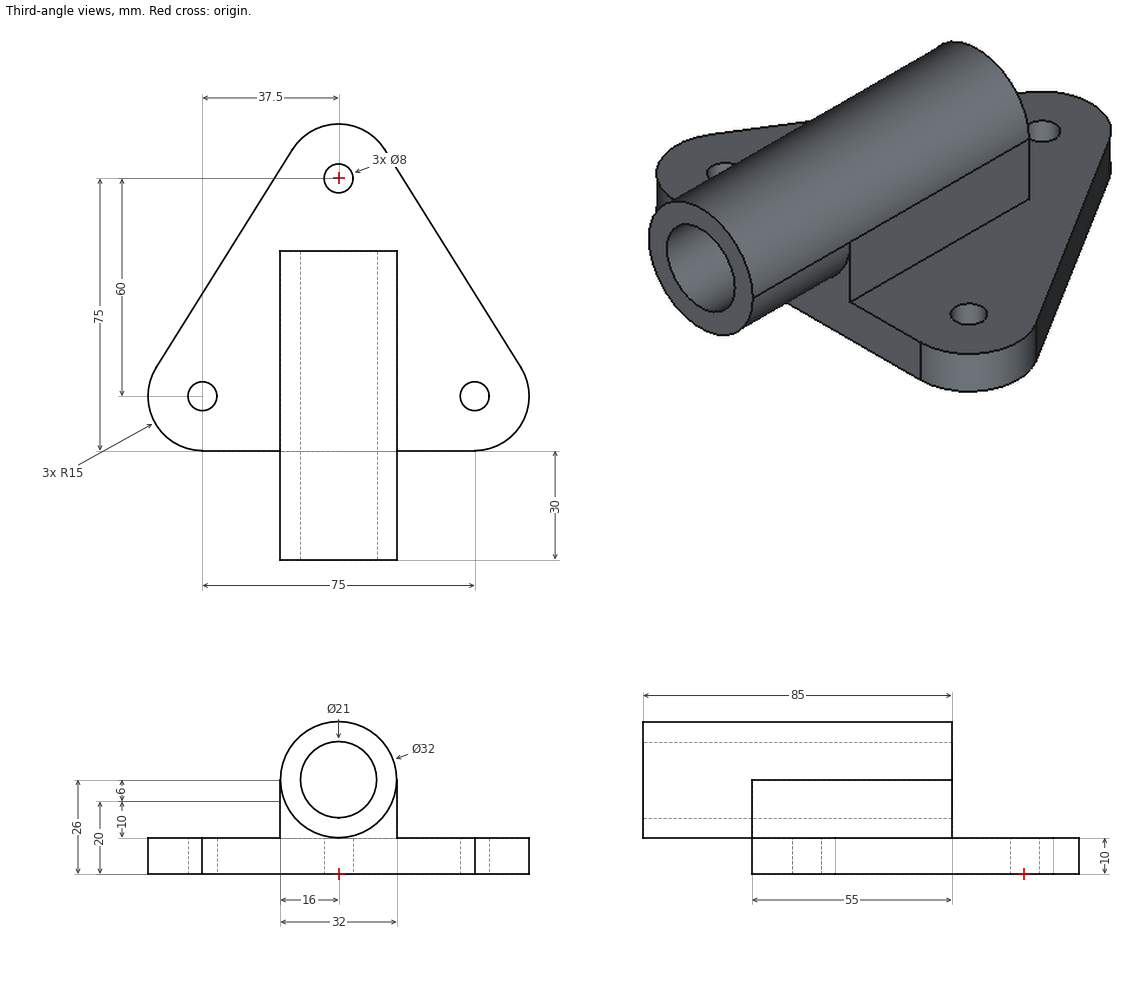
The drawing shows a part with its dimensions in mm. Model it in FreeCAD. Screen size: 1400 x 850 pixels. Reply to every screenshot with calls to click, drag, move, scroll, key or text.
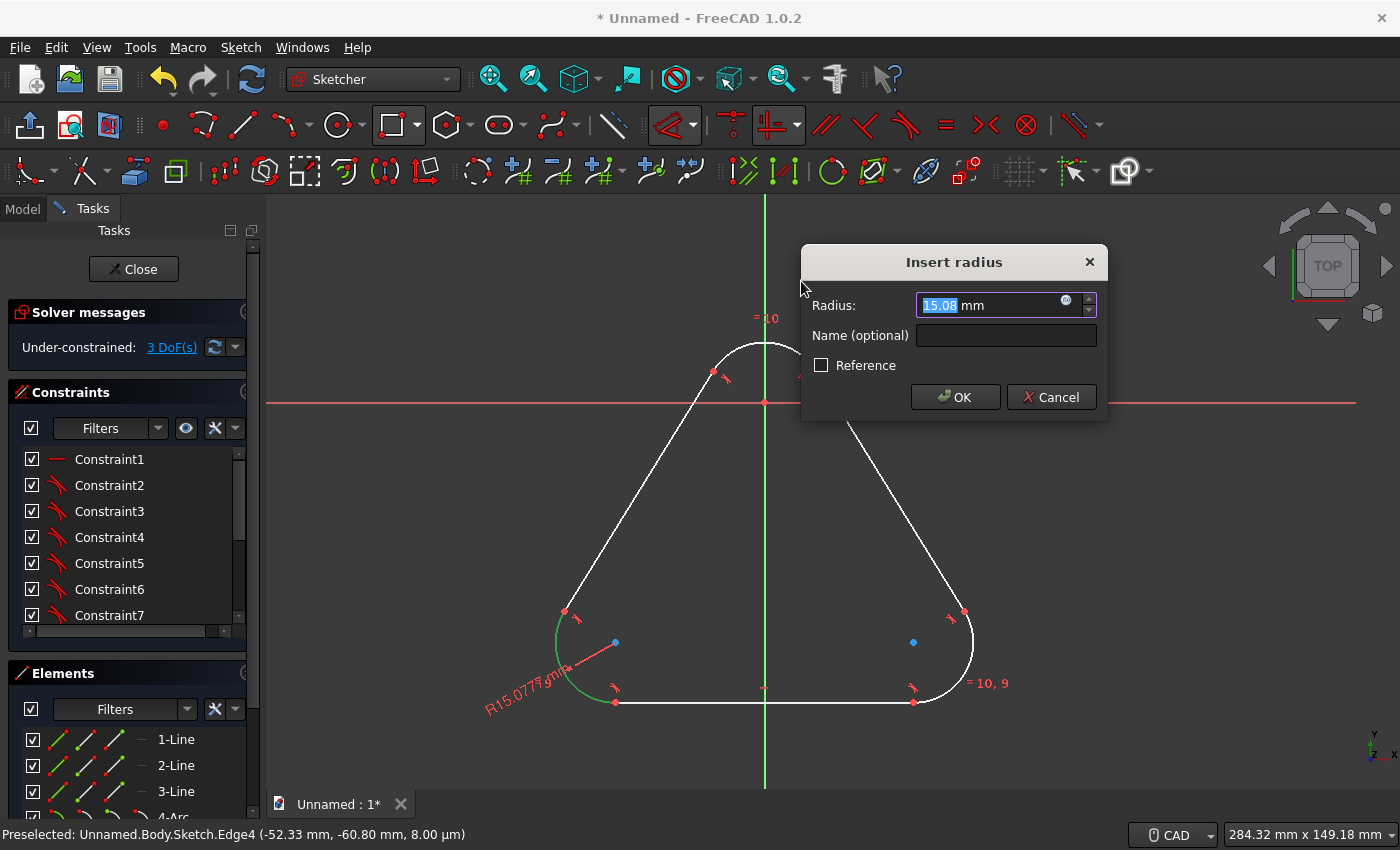
text(15)
key(Return)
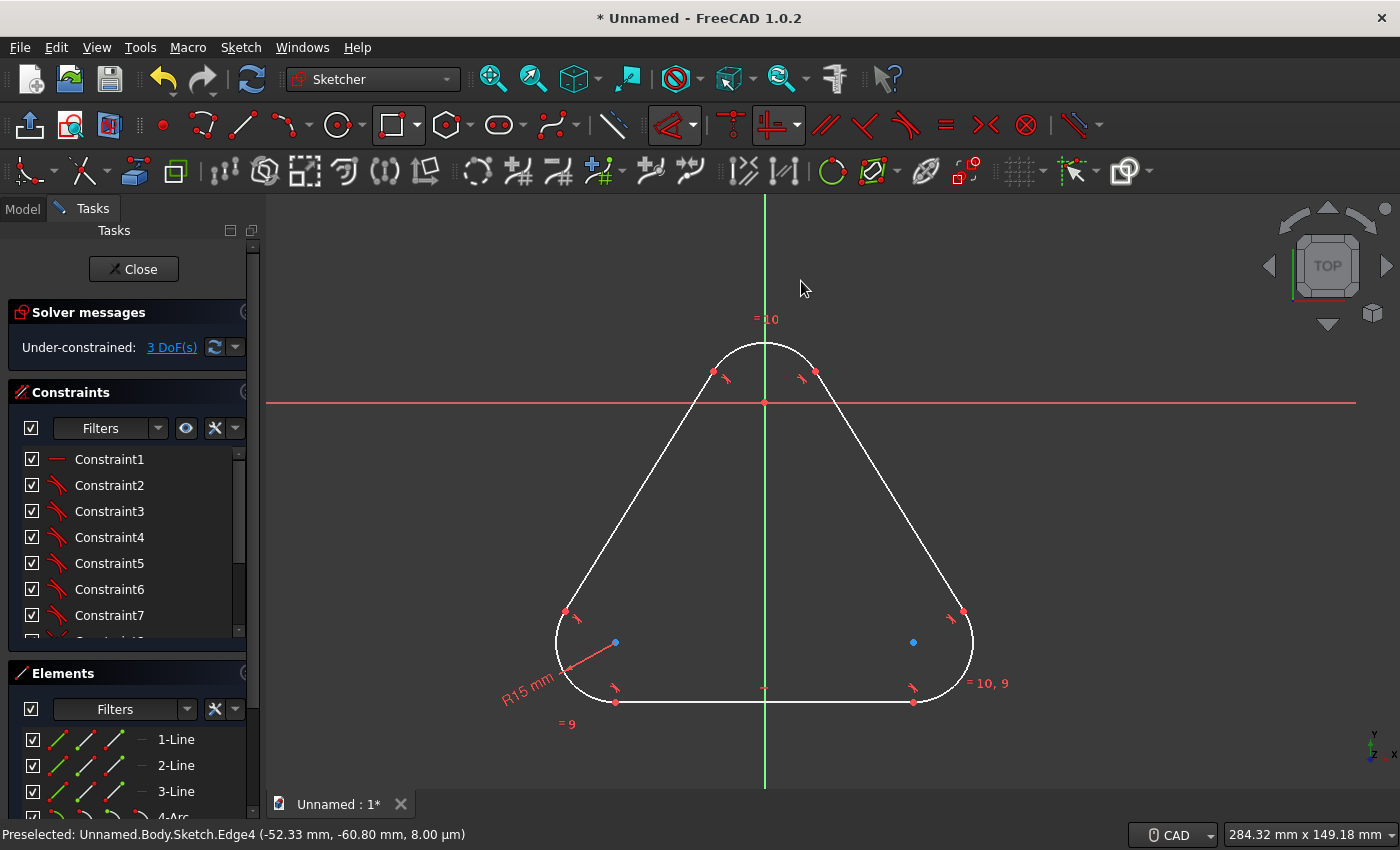
click(705, 702)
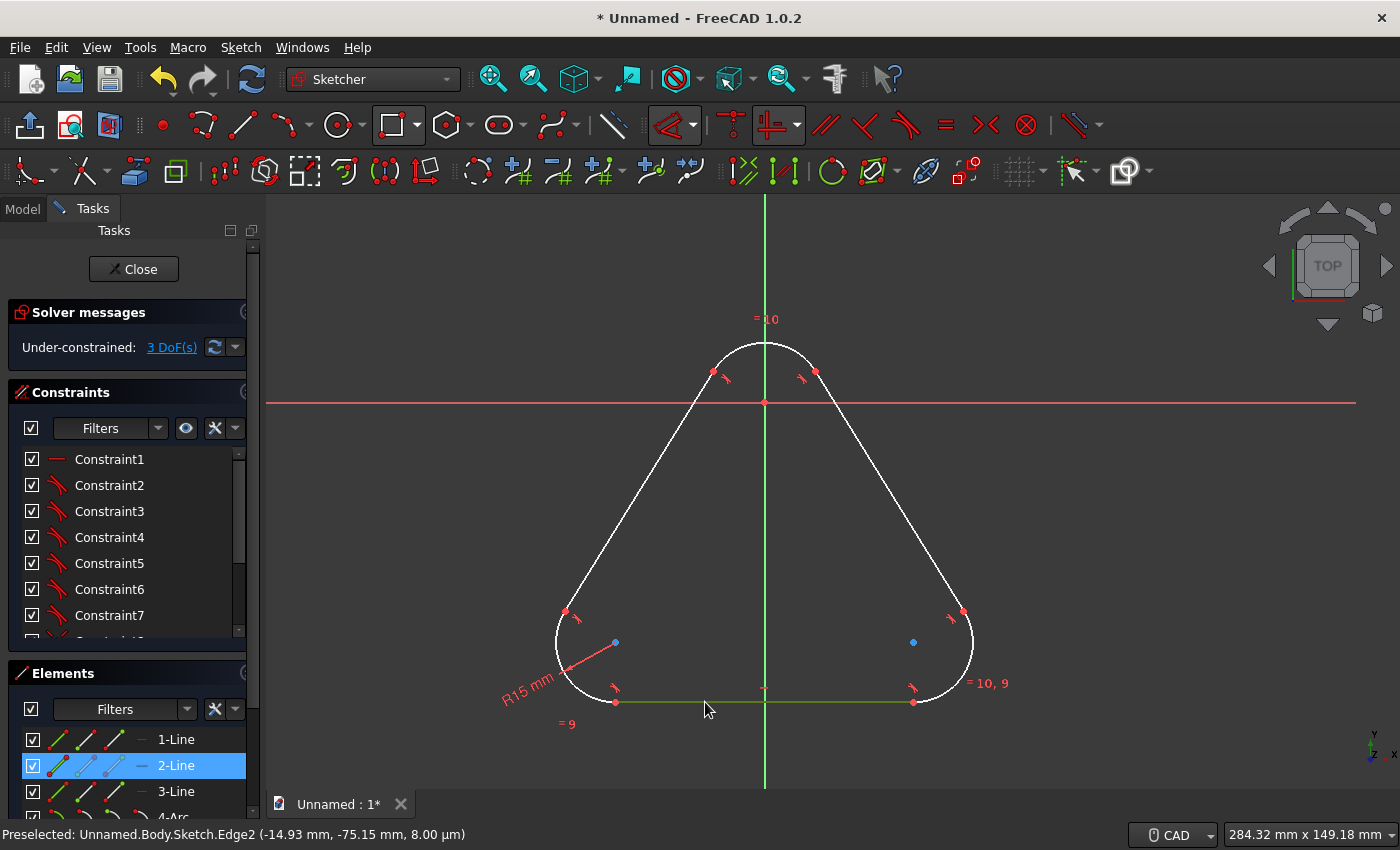
click(696, 126)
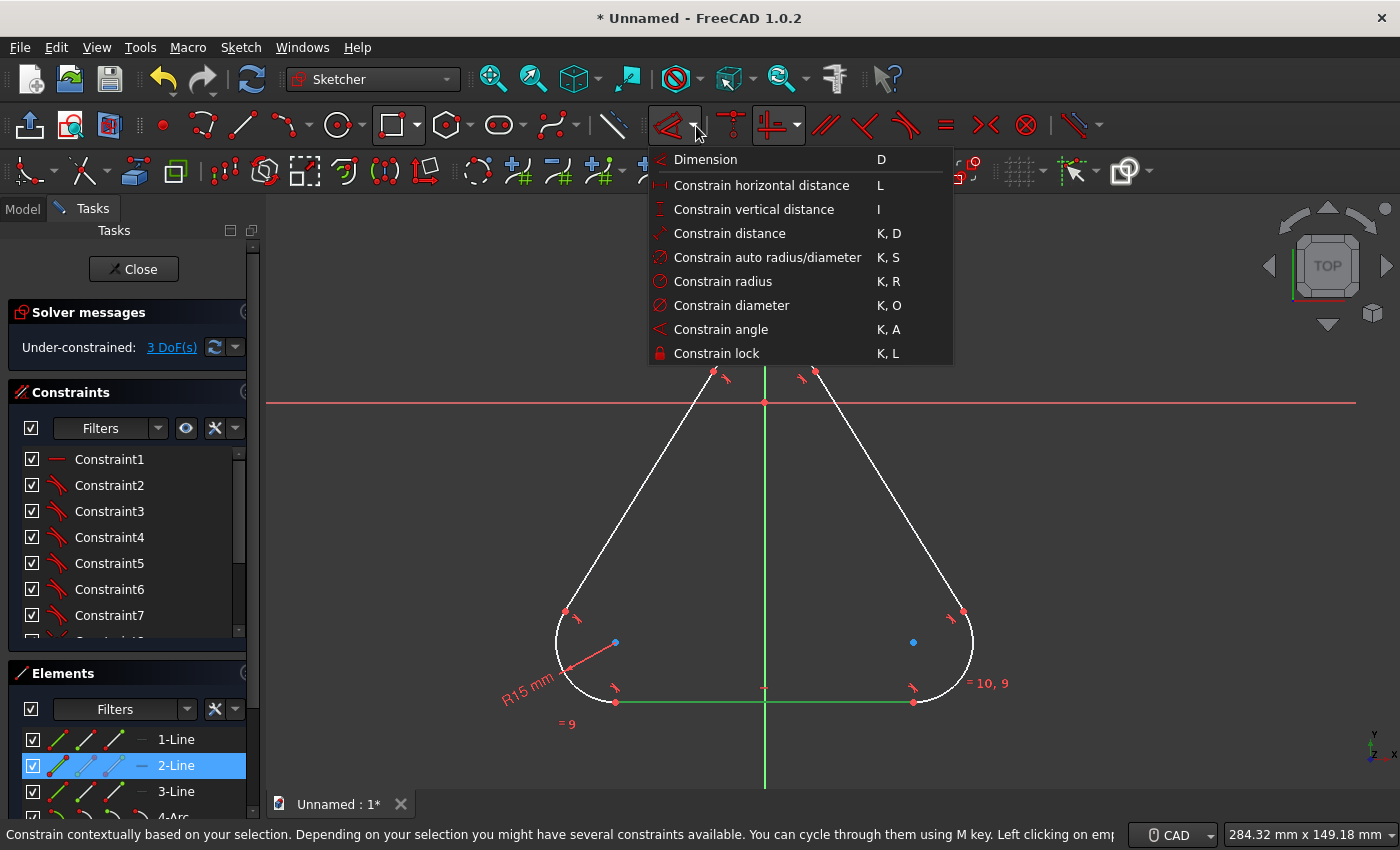
click(801, 185)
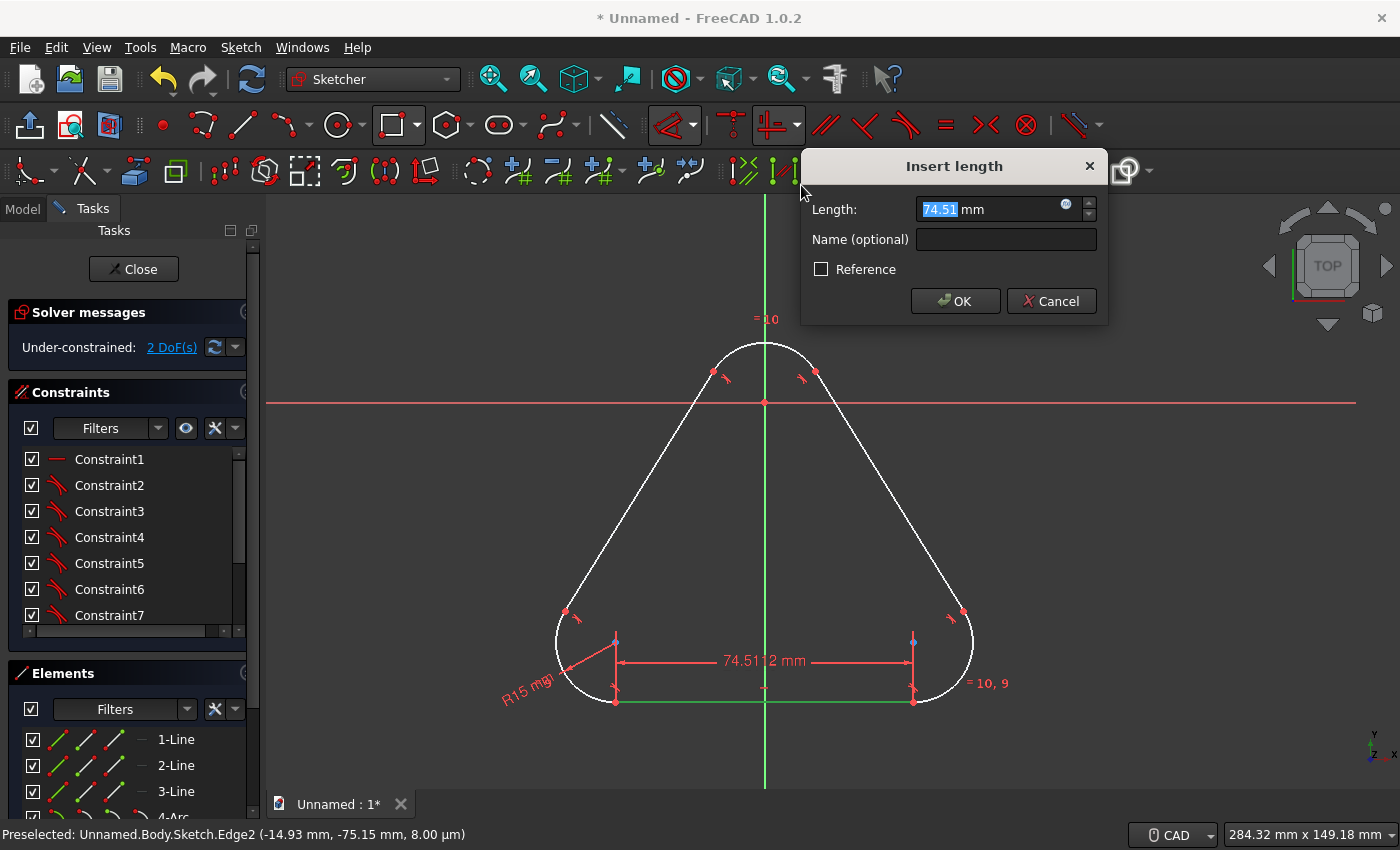
text(75)
key(Return)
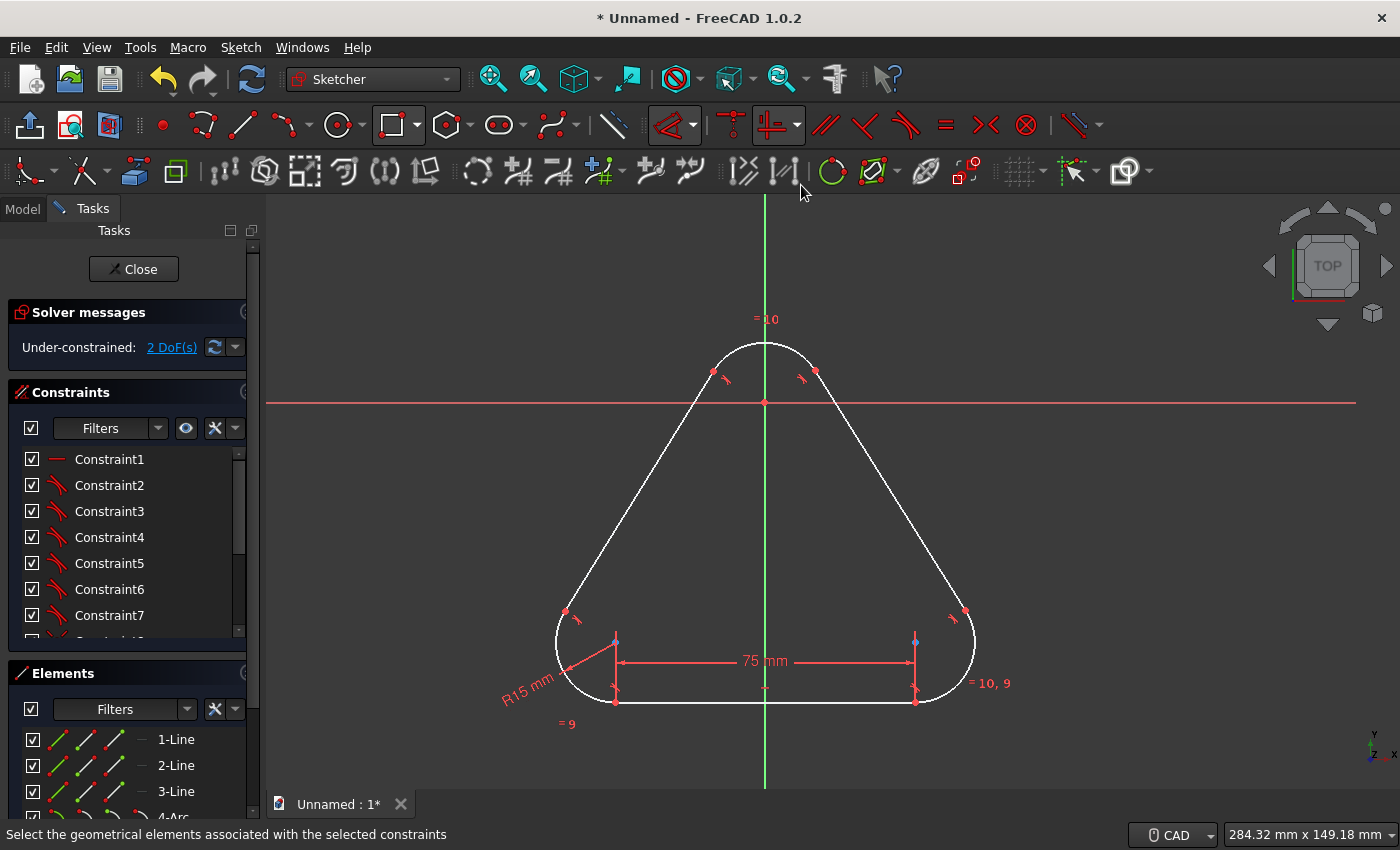
click(616, 703)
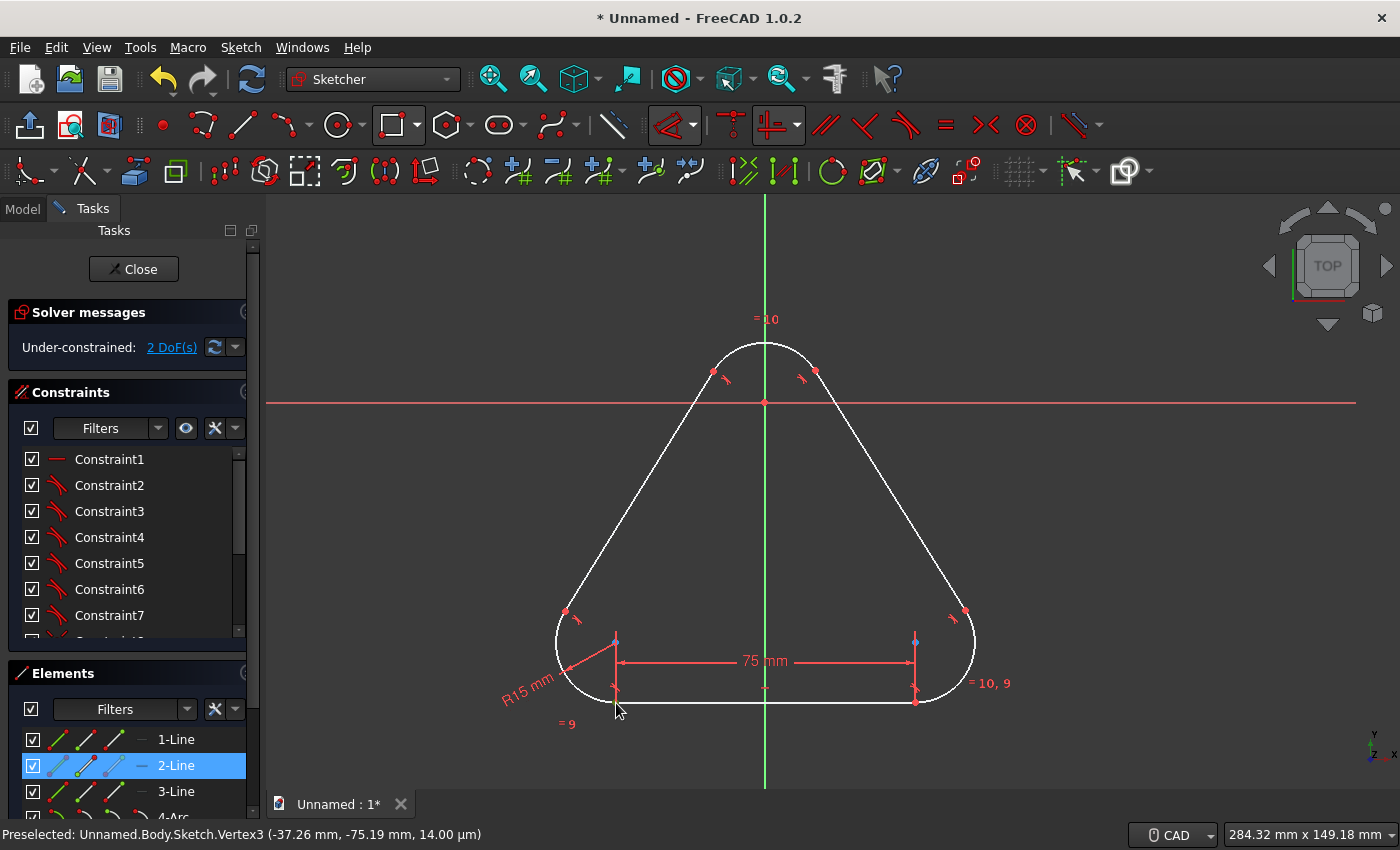
click(696, 126)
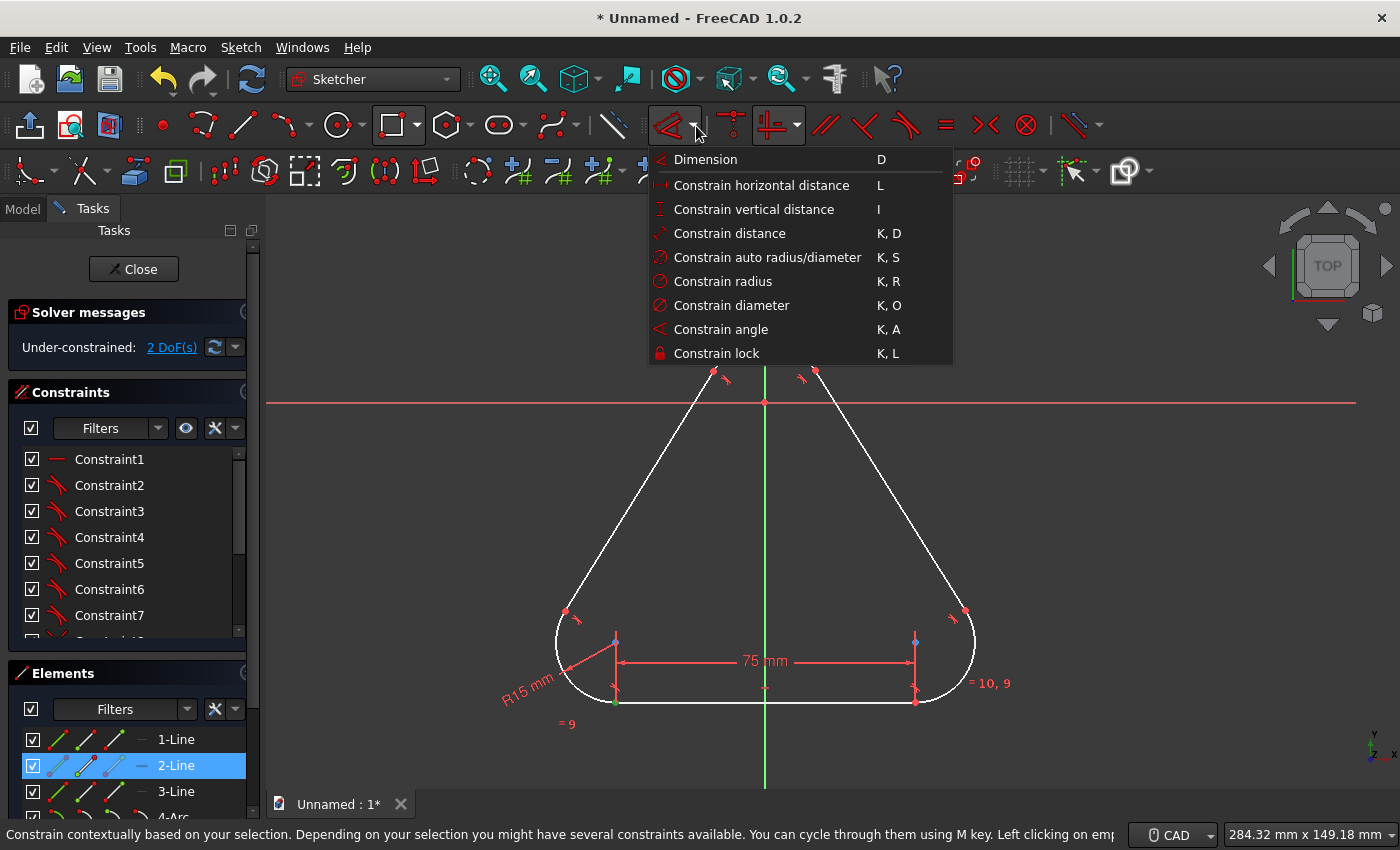
click(801, 209)